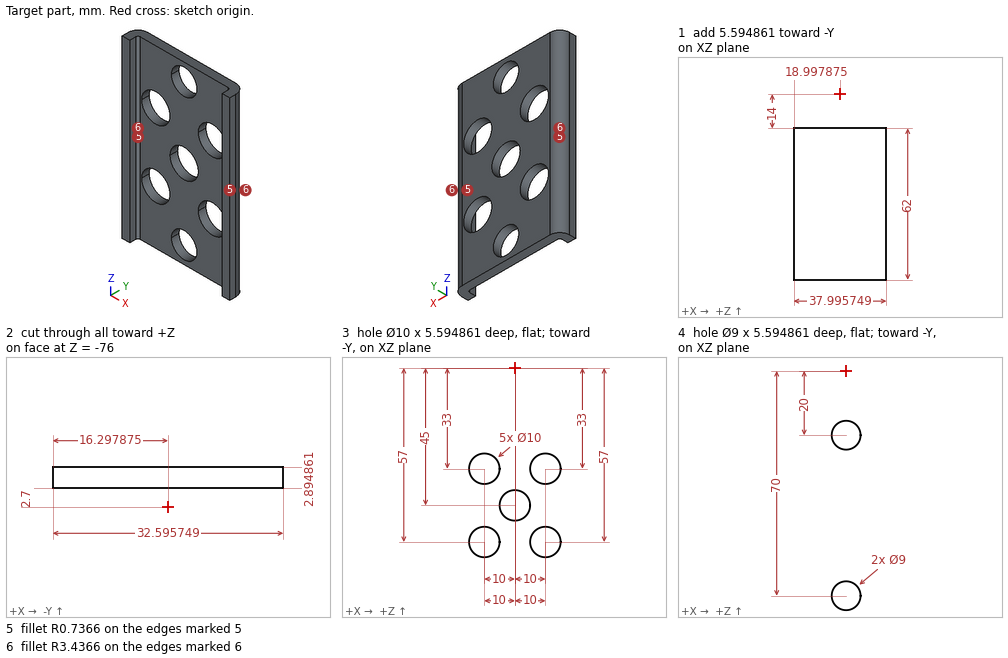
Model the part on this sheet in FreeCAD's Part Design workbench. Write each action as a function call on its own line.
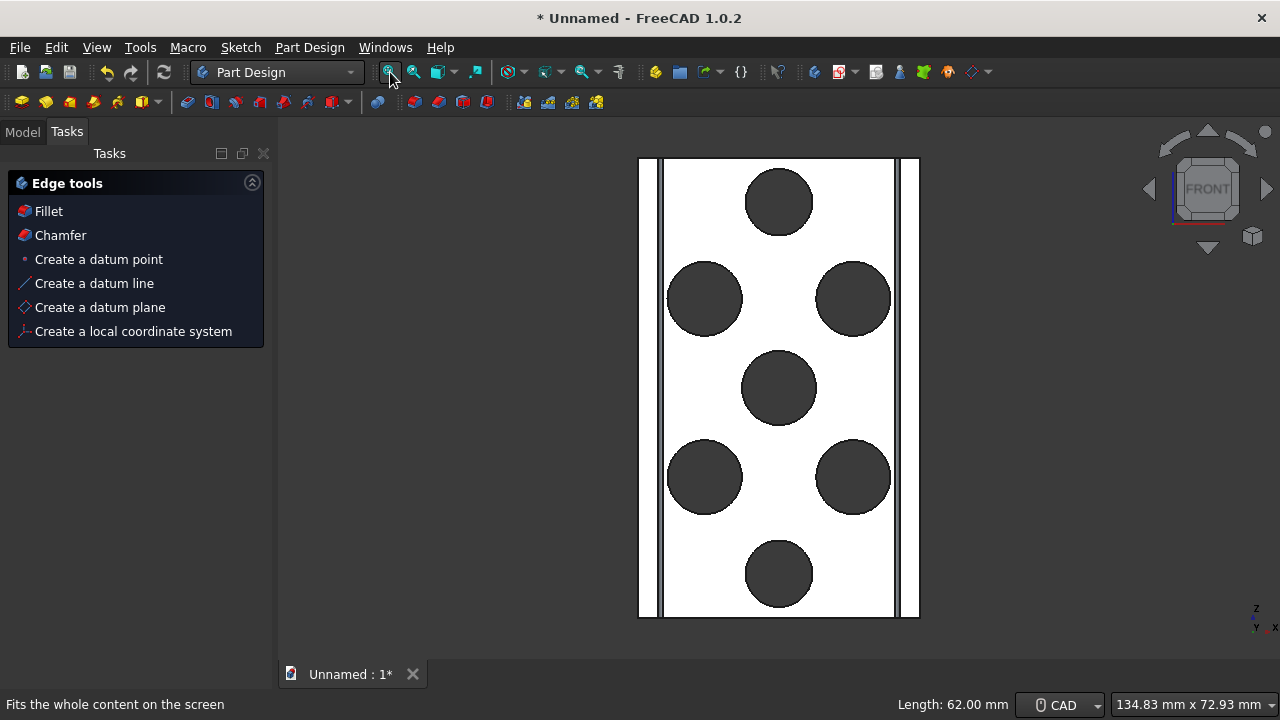
key(3)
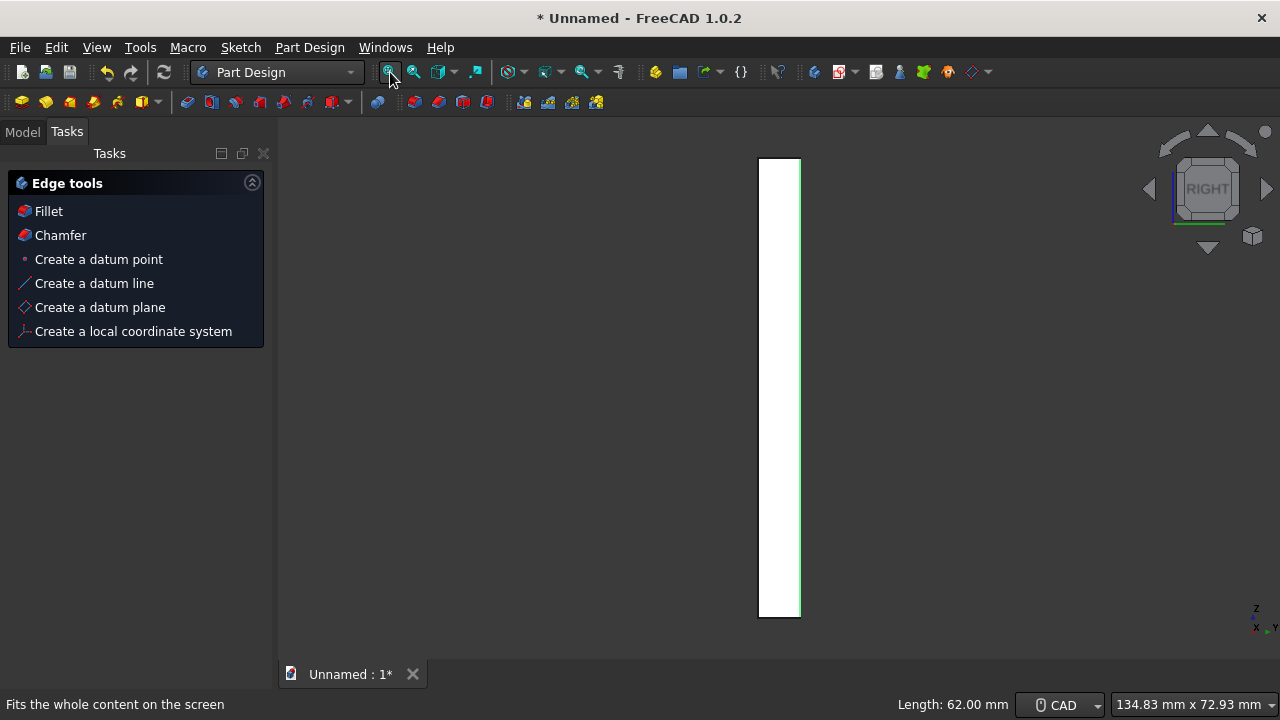
key(5)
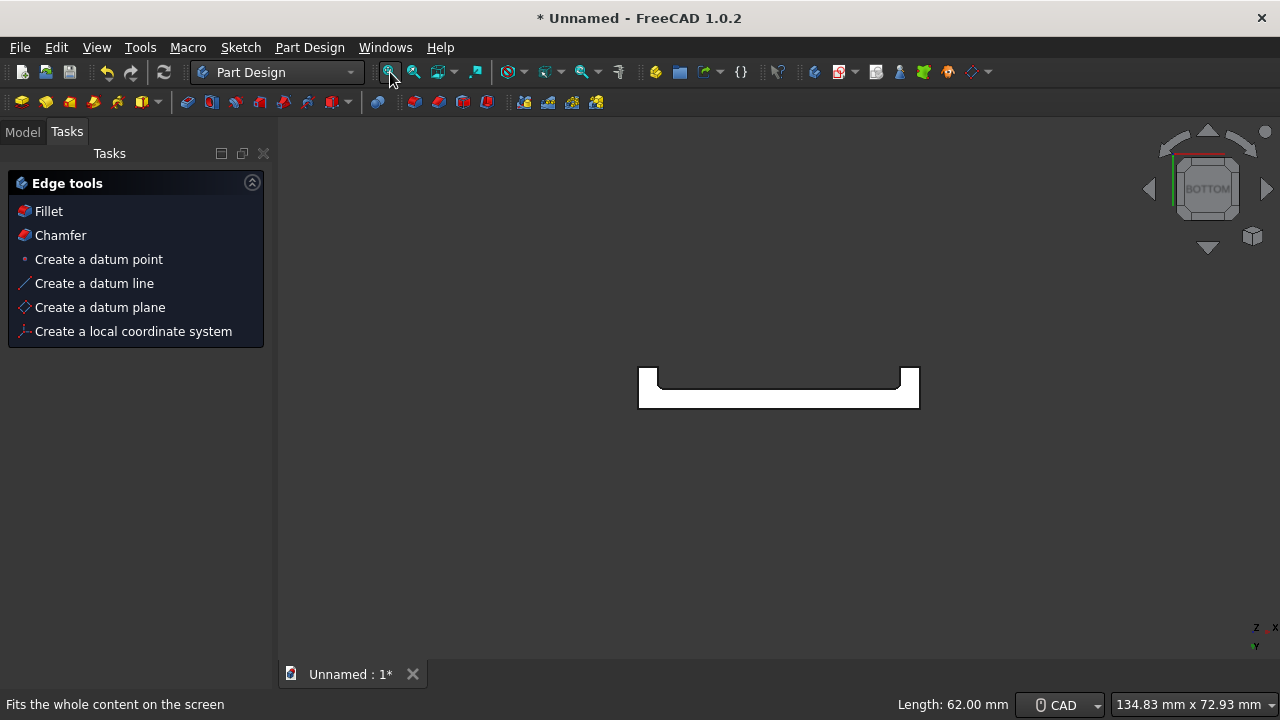
click(390, 72)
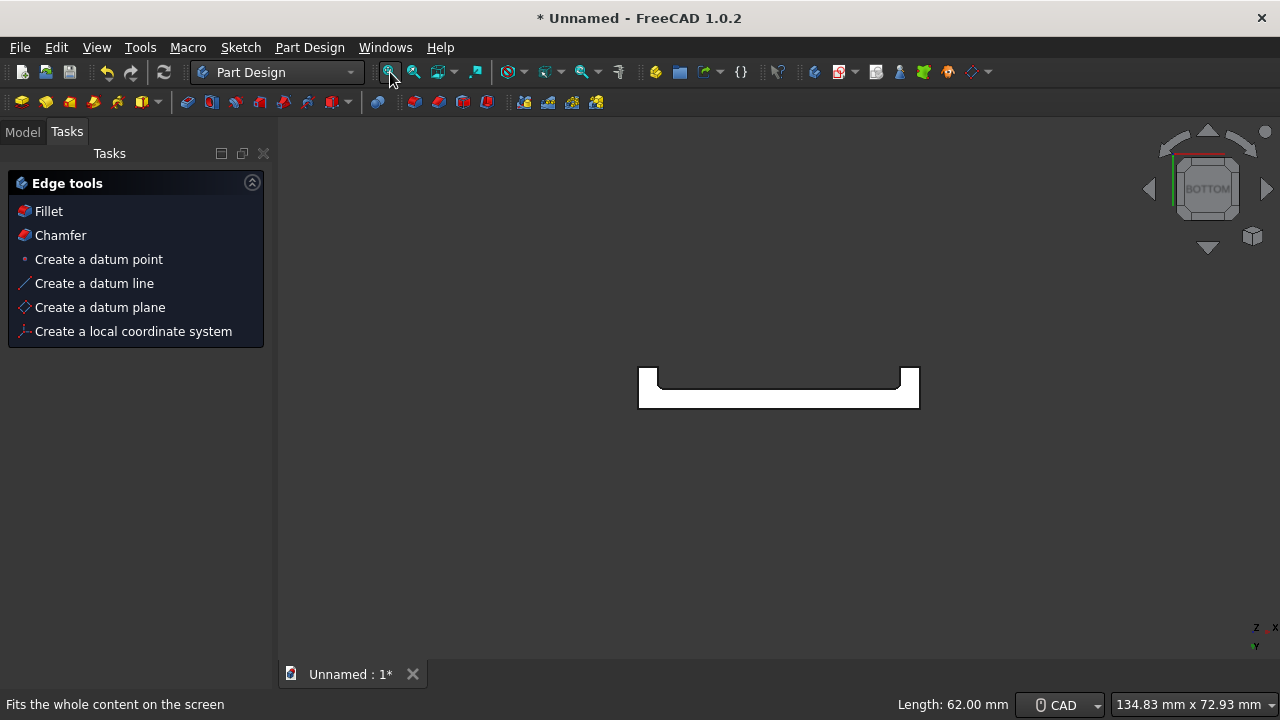
key(4)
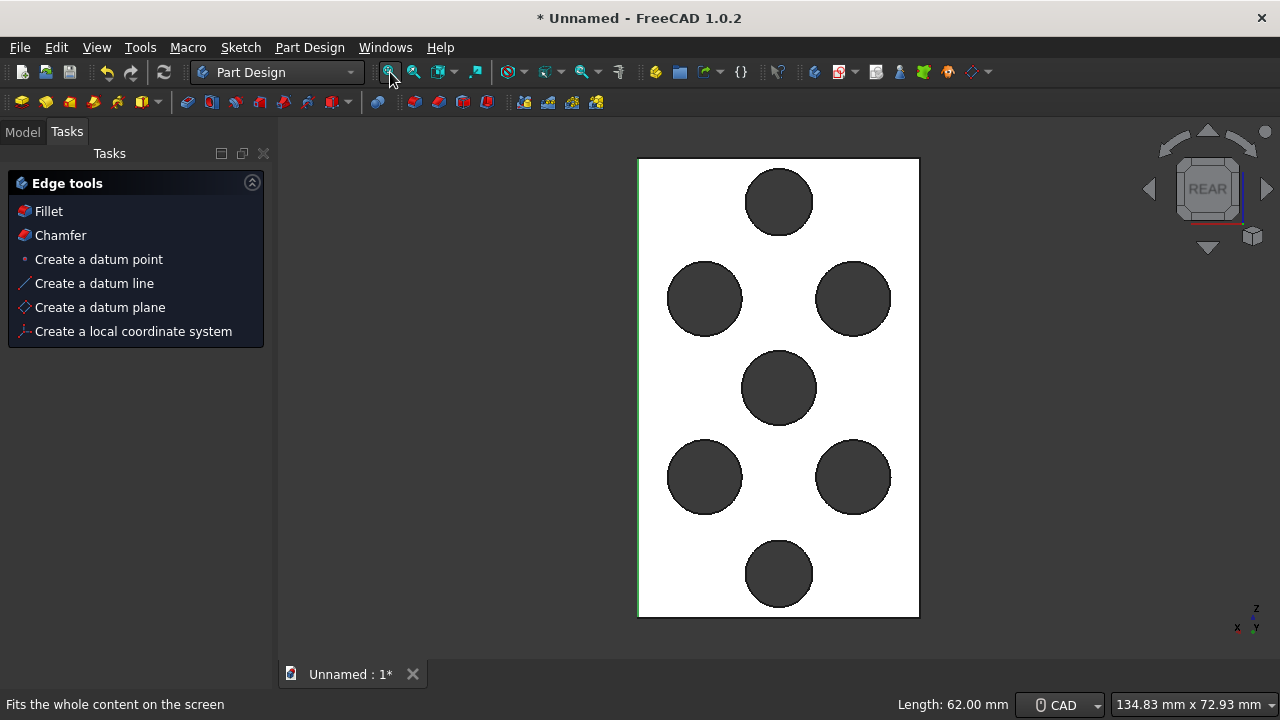
click(920, 387, ctrl)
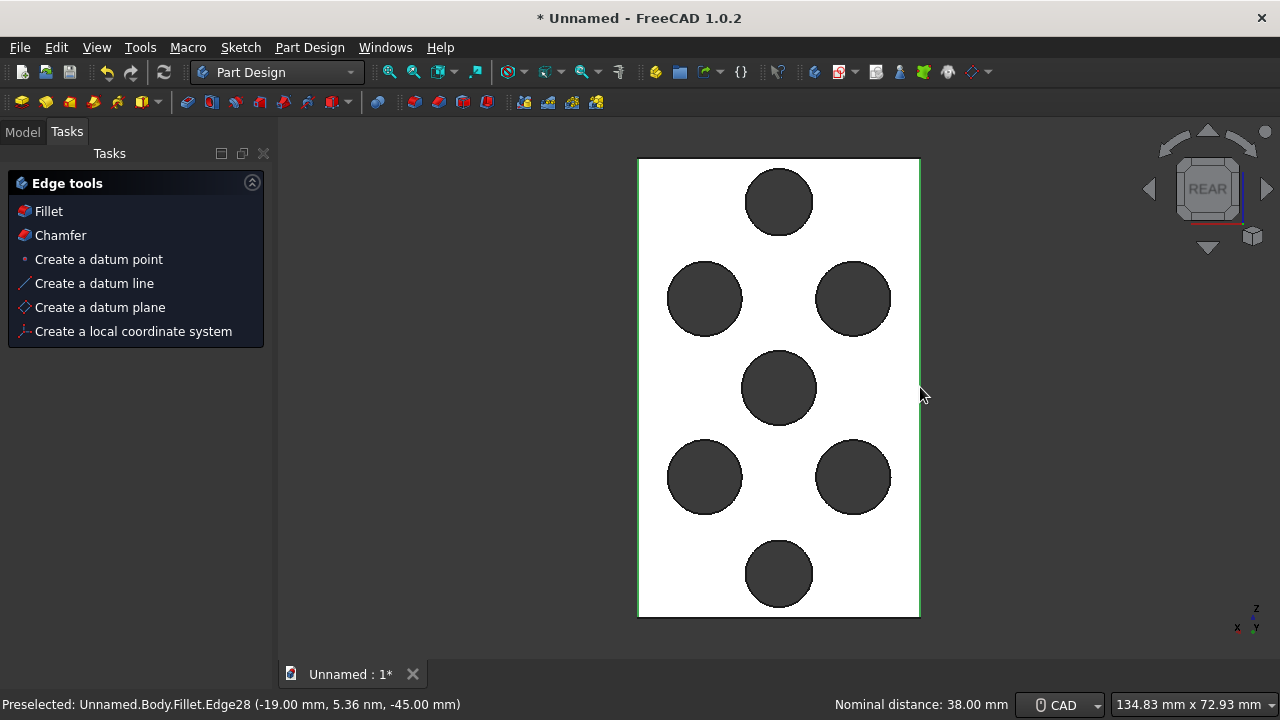
click(416, 102)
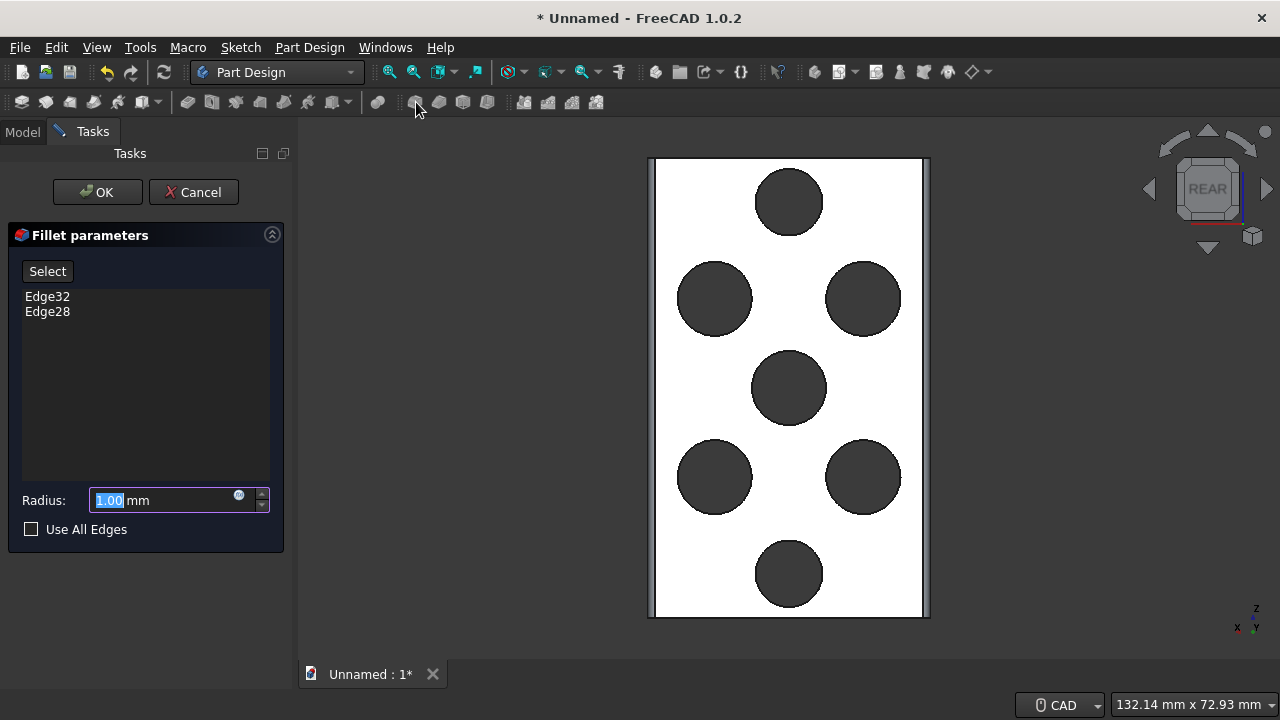
text(3.4366)
key(Tab)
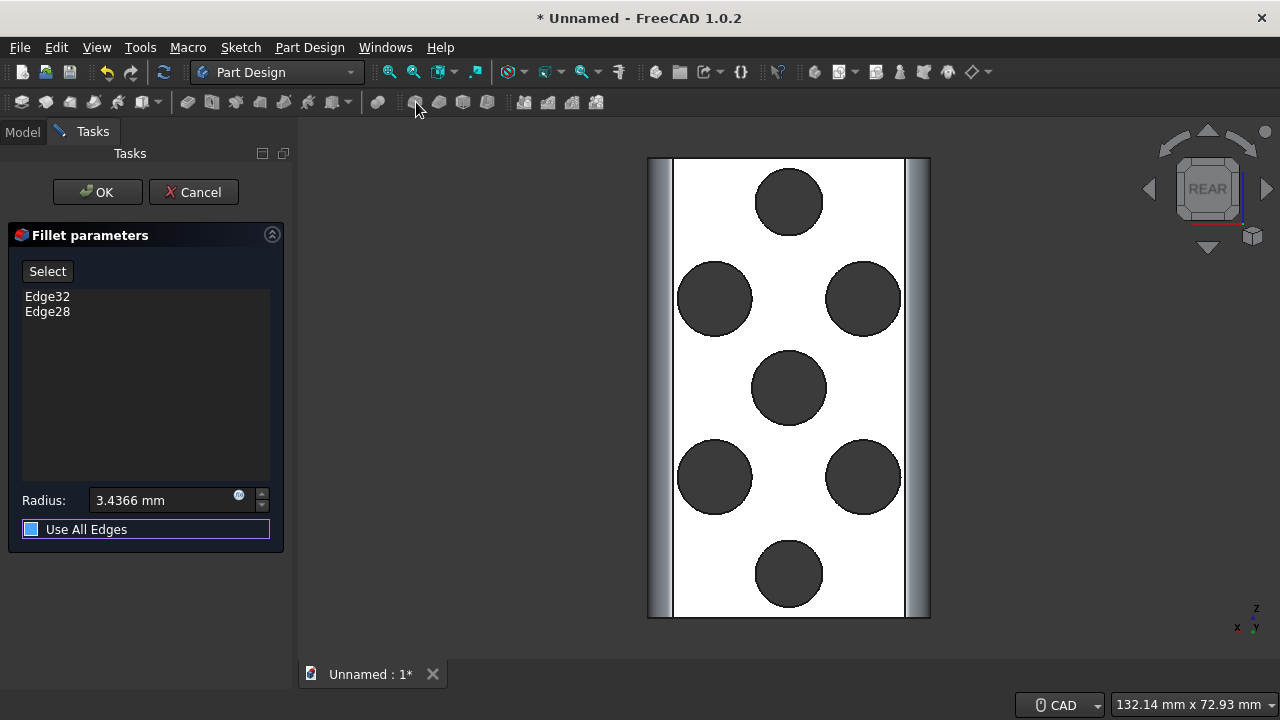
click(98, 192)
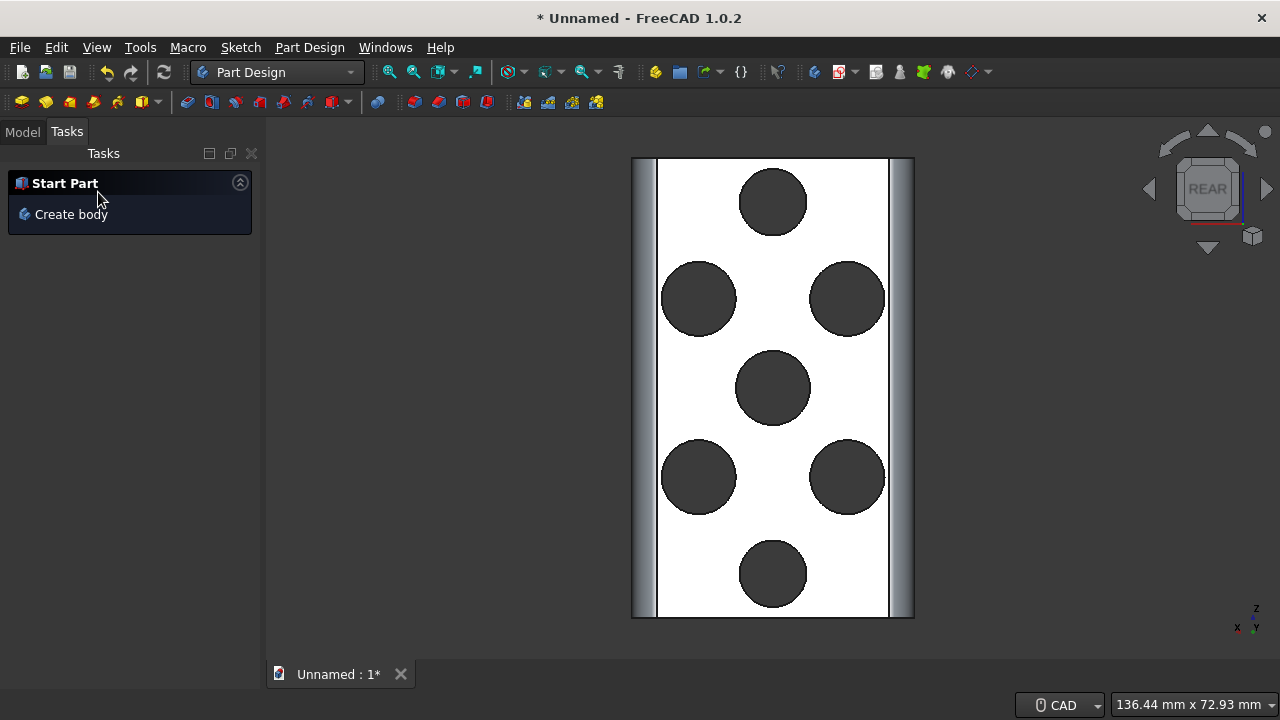
key(0)